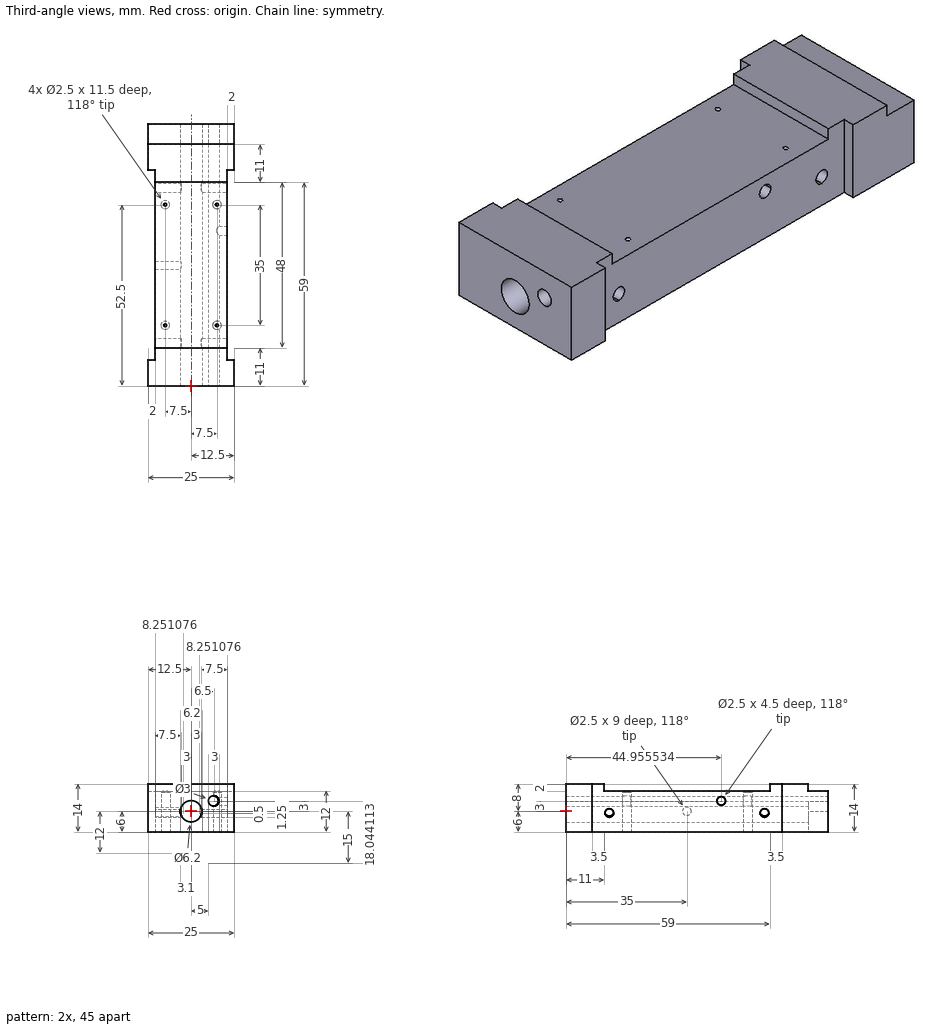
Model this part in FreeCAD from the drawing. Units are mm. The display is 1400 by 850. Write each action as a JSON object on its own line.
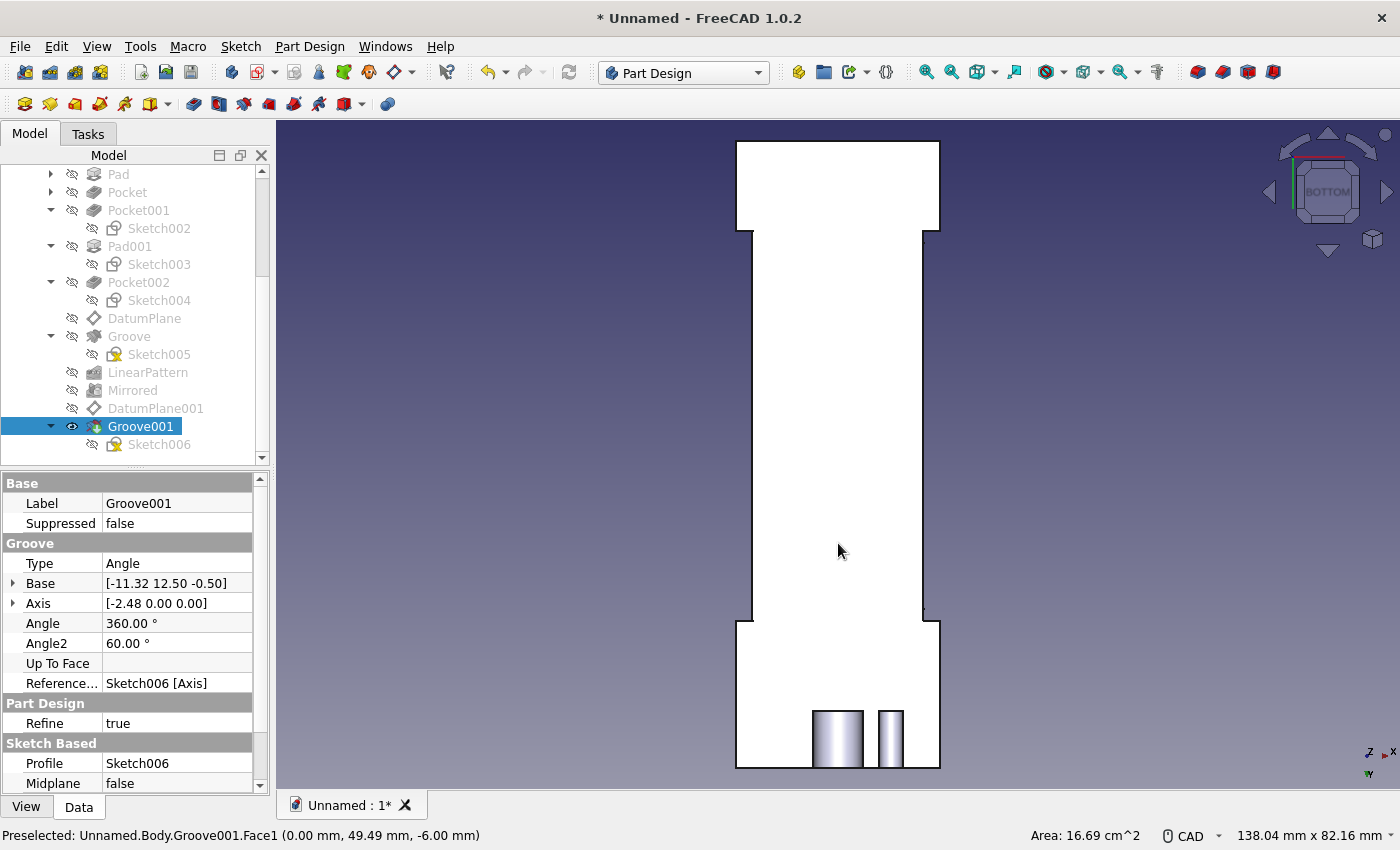
{"action": "left_click", "coordinate": [256, 72]}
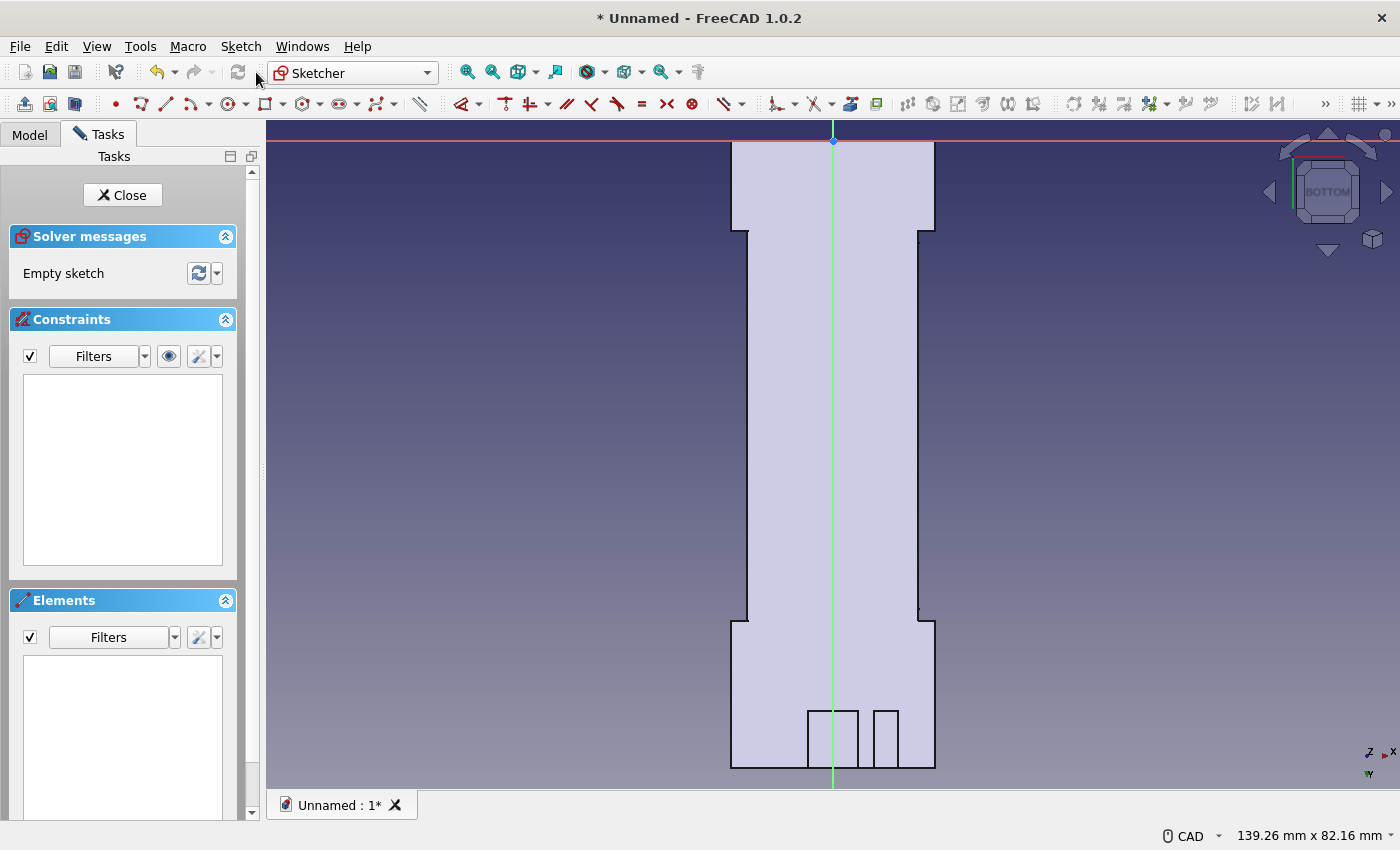
{"action": "scroll", "coordinate": [455, 761], "scroll_direction": "down", "scroll_amount": 1}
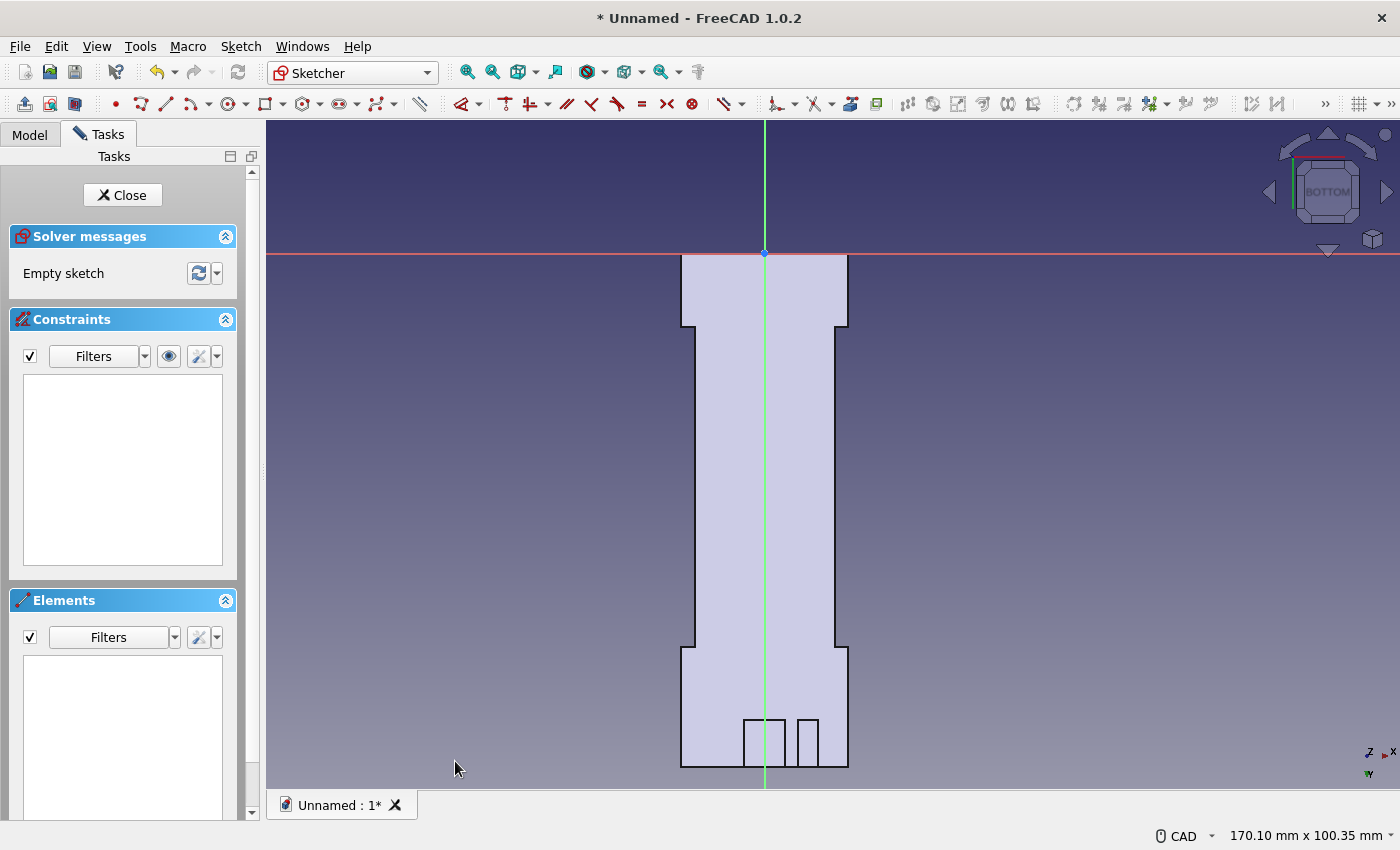
{"action": "left_click", "coordinate": [228, 104]}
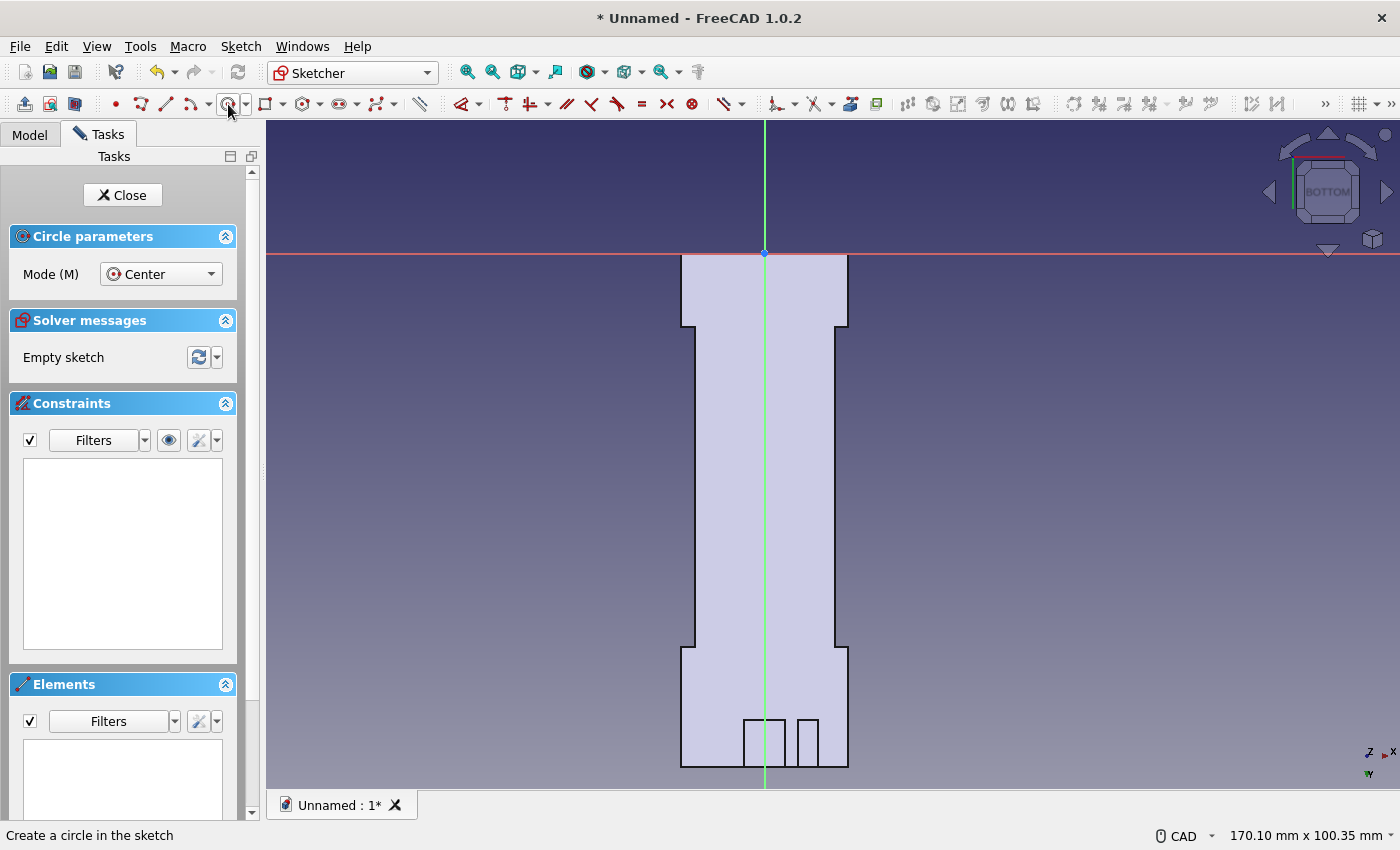
{"action": "scroll", "coordinate": [715, 604], "scroll_direction": "up", "scroll_amount": 6}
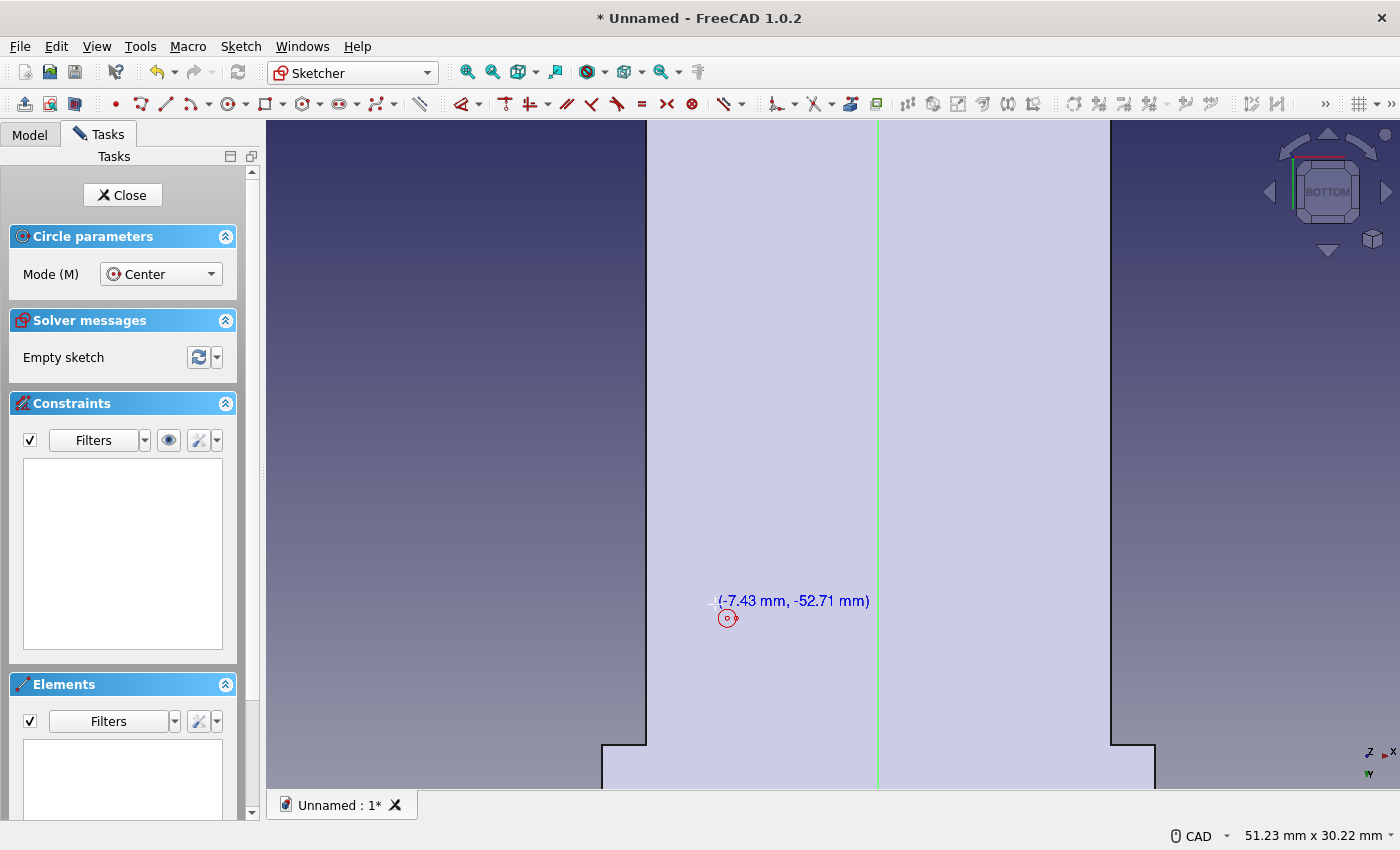
{"action": "left_click", "coordinate": [712, 601]}
{"action": "left_click", "coordinate": [732, 581]}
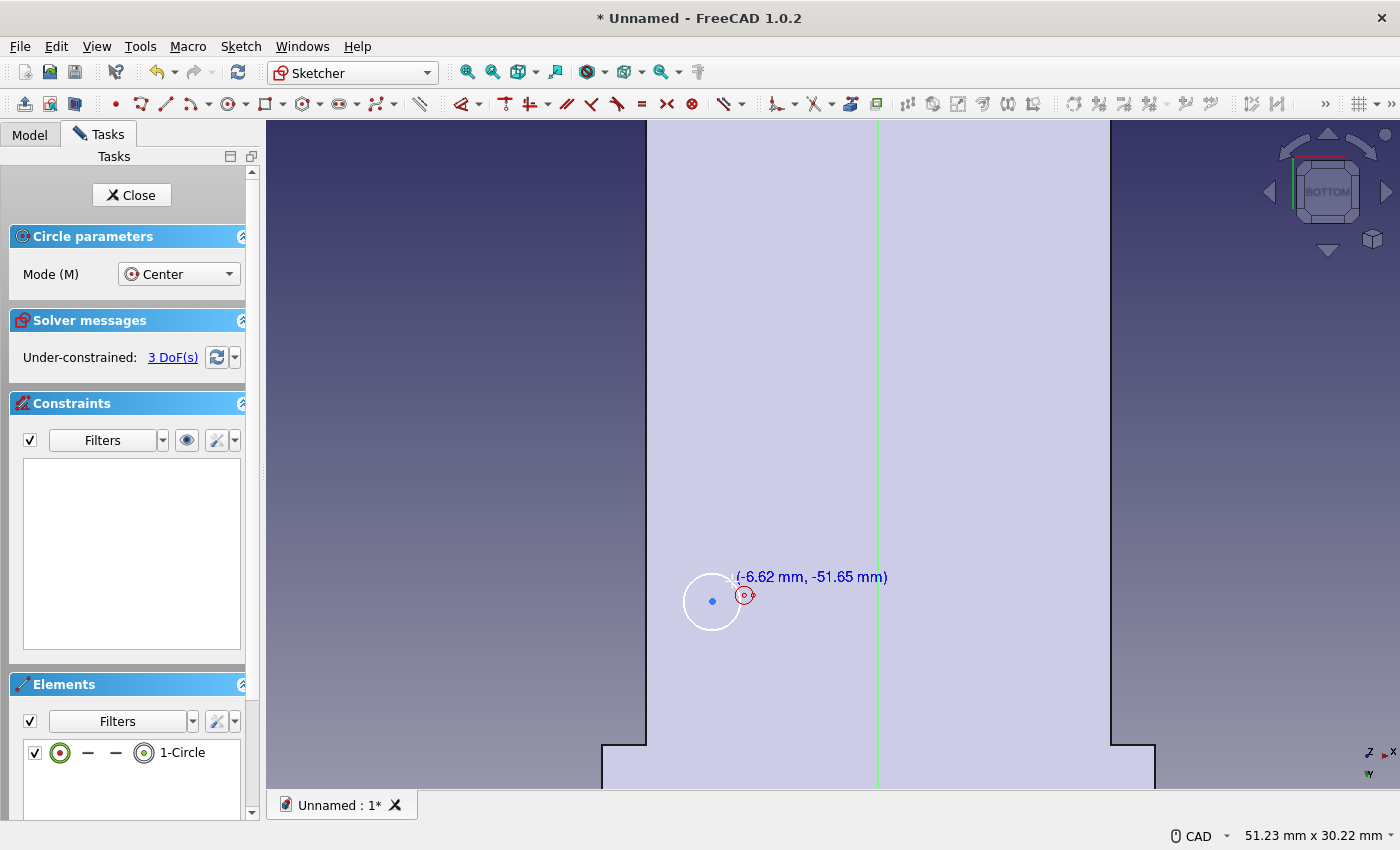
{"action": "left_click", "coordinate": [1044, 601]}
{"action": "left_click", "coordinate": [1064, 581]}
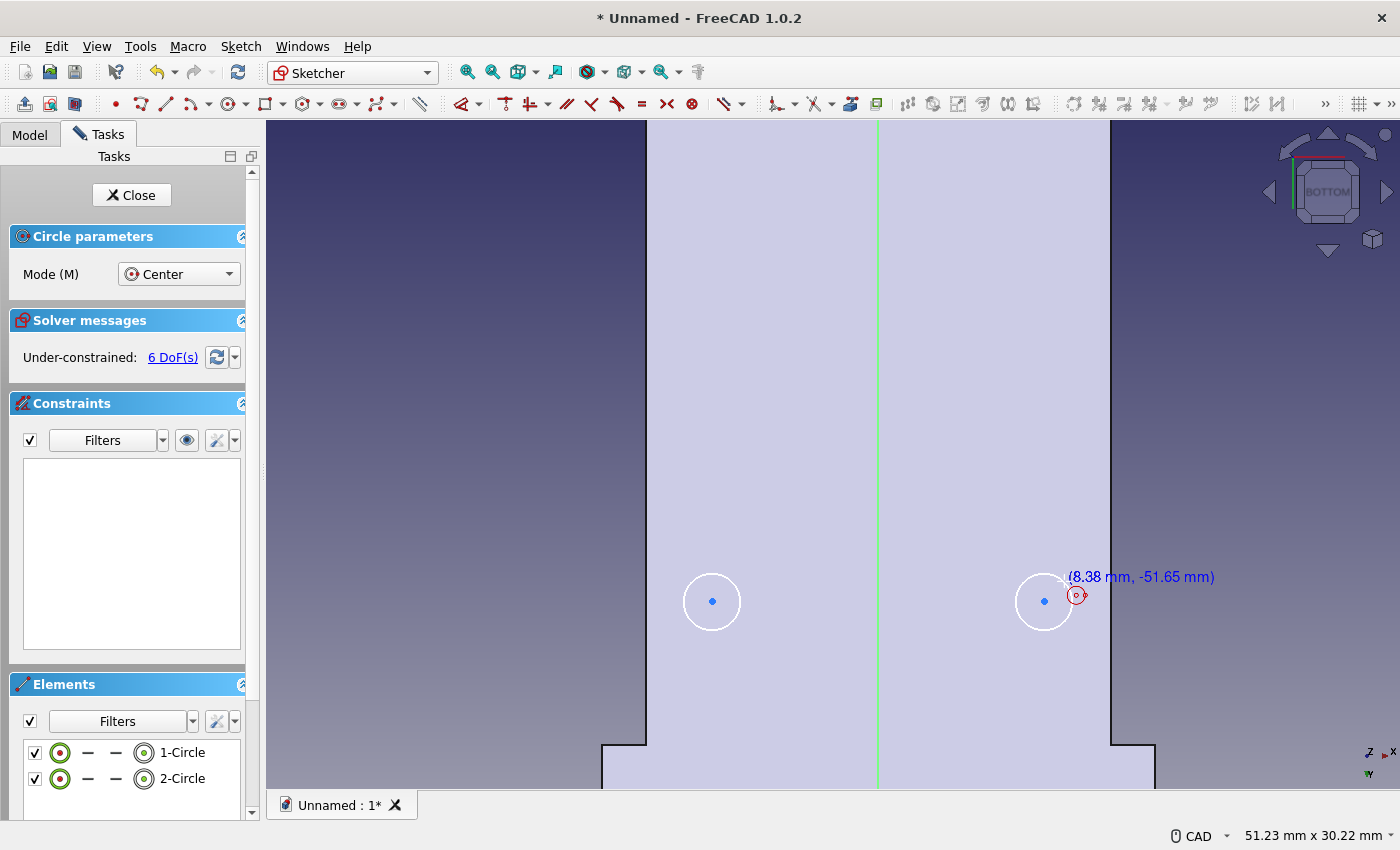
{"action": "scroll", "coordinate": [698, 699], "scroll_direction": "down", "scroll_amount": 5}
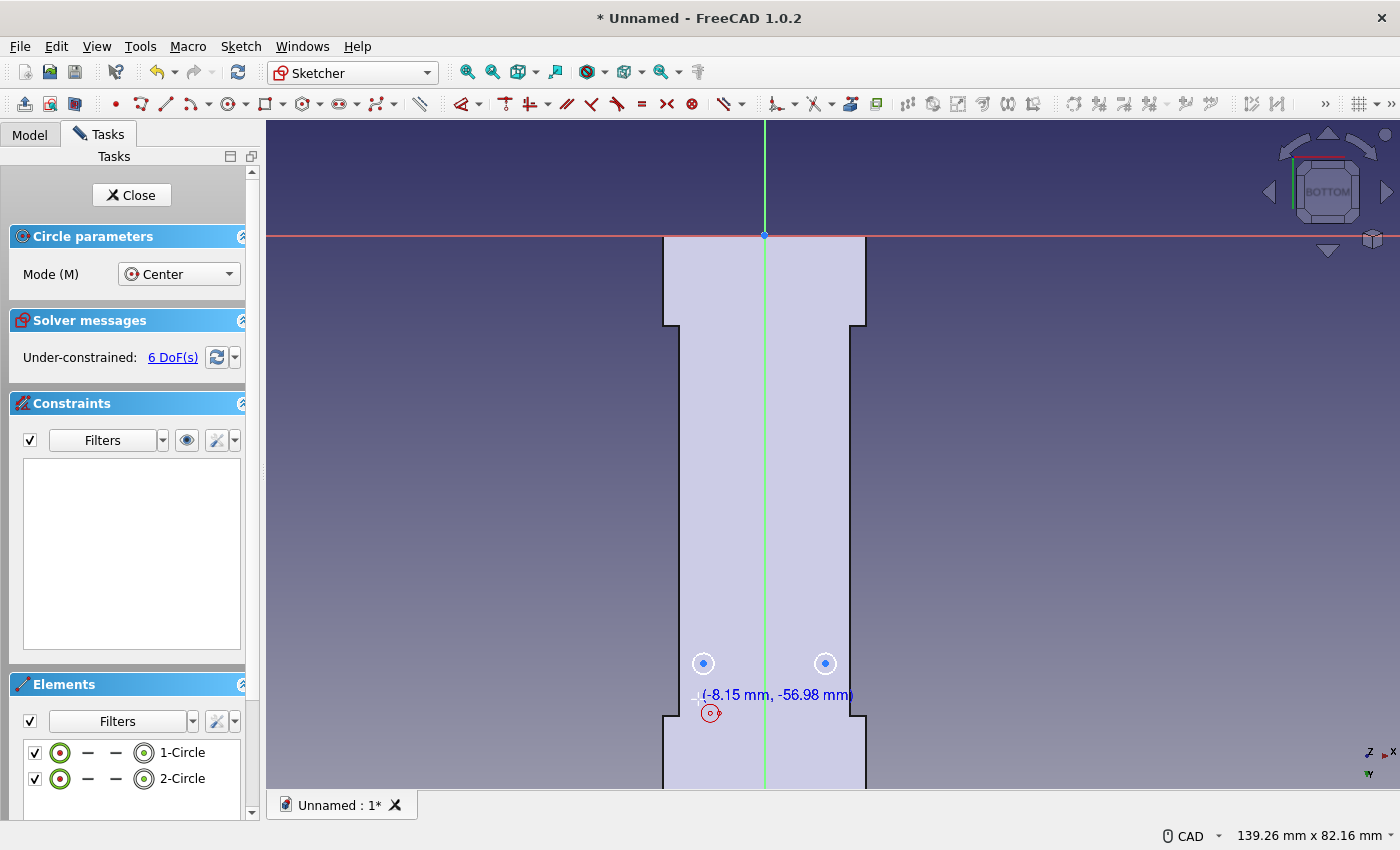
{"action": "scroll", "coordinate": [826, 378], "scroll_direction": "up", "scroll_amount": 5}